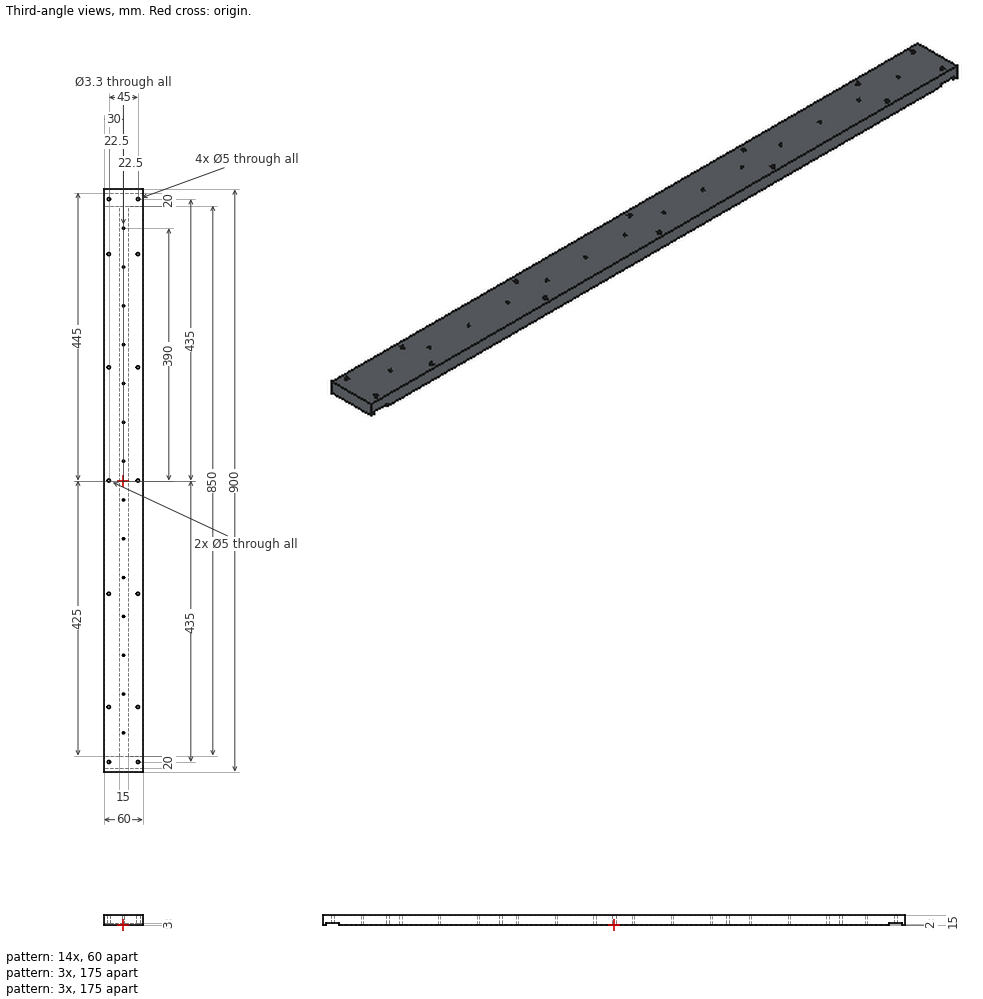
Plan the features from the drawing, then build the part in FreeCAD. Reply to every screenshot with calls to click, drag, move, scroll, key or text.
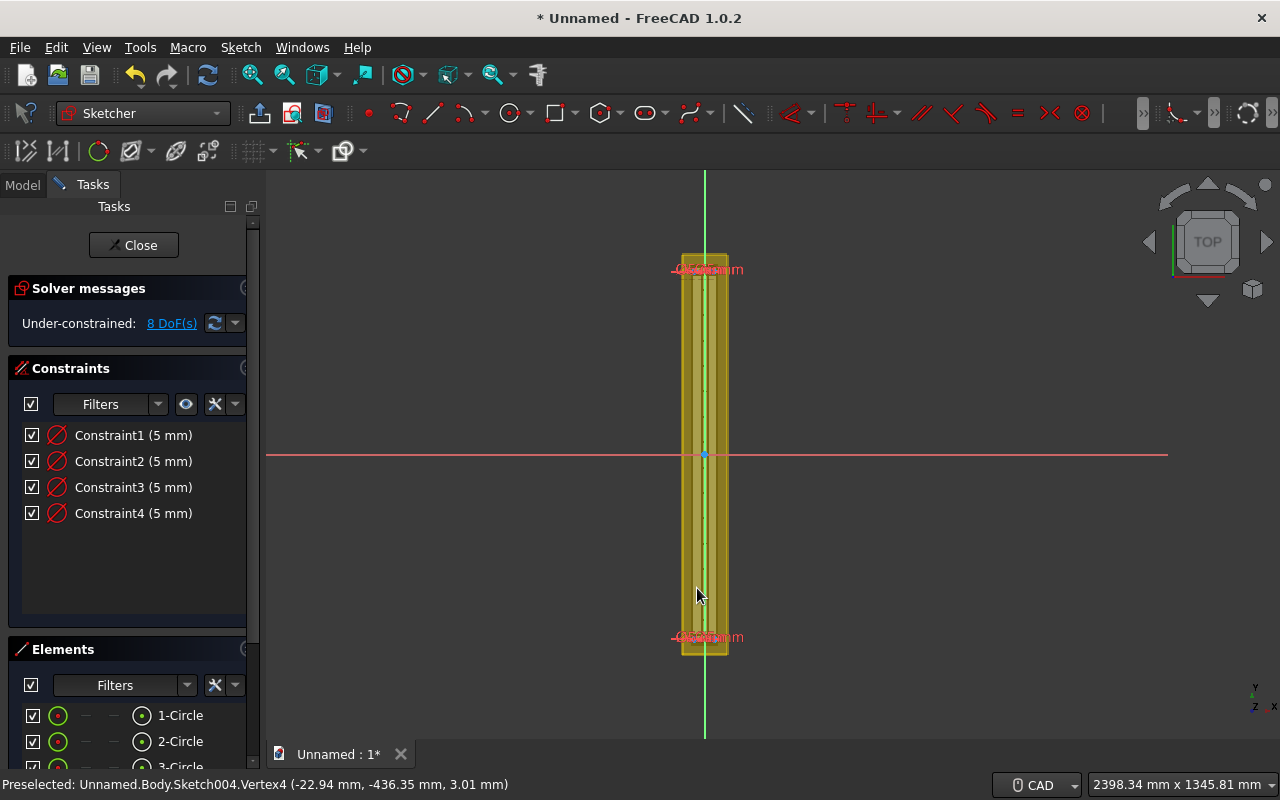
click(714, 272)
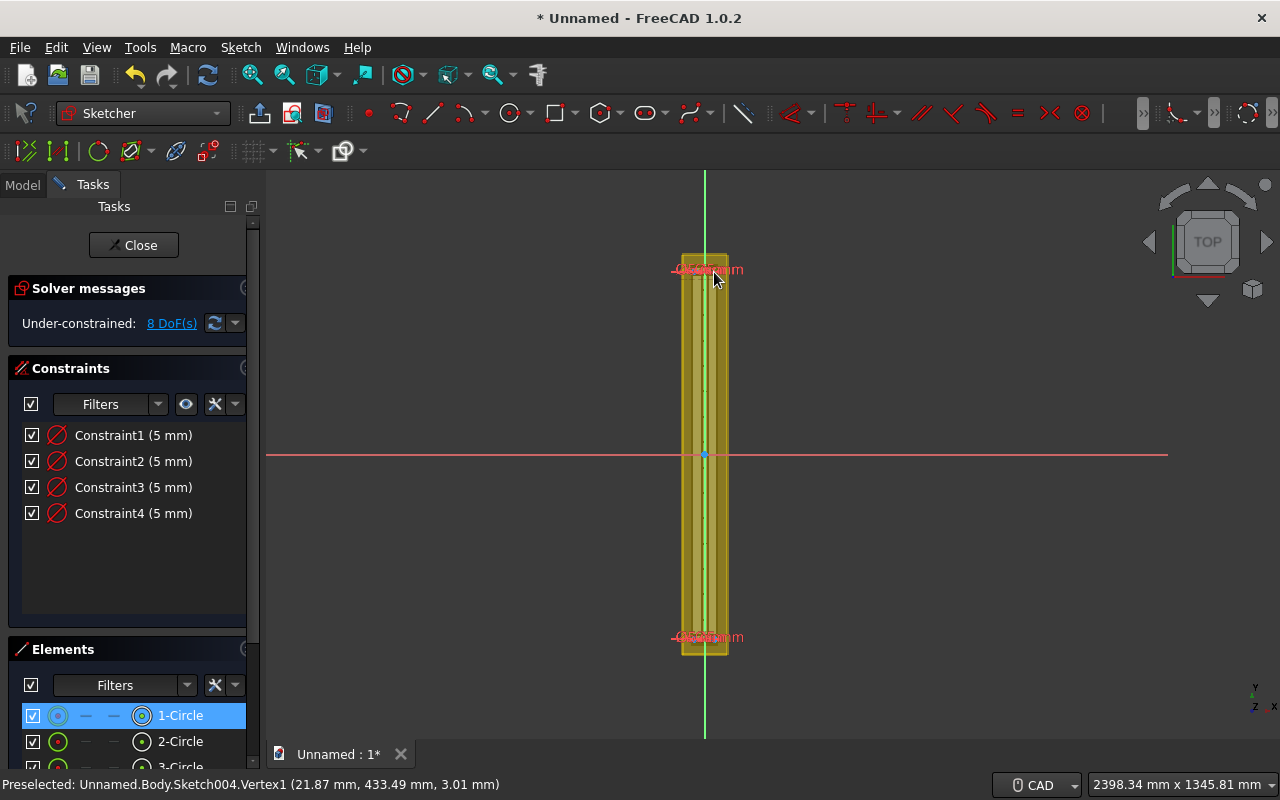
click(695, 272)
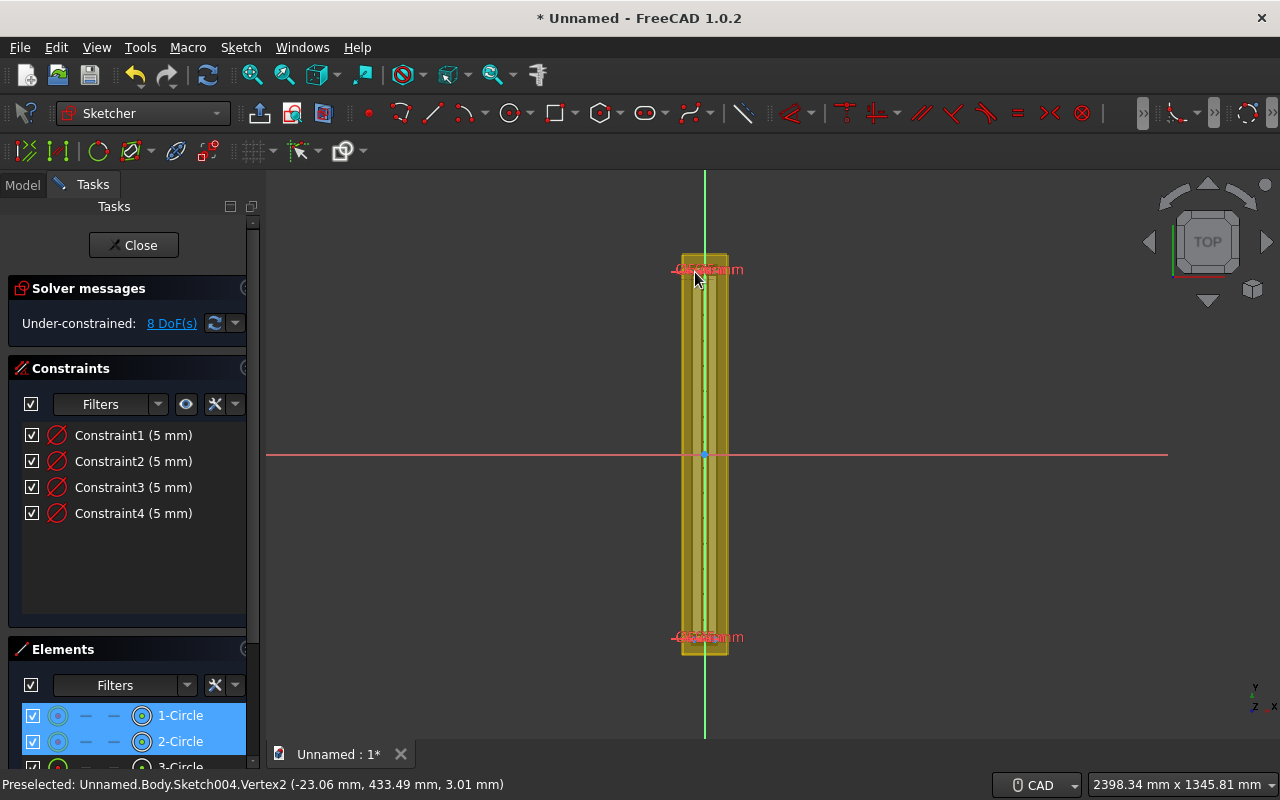
key(h)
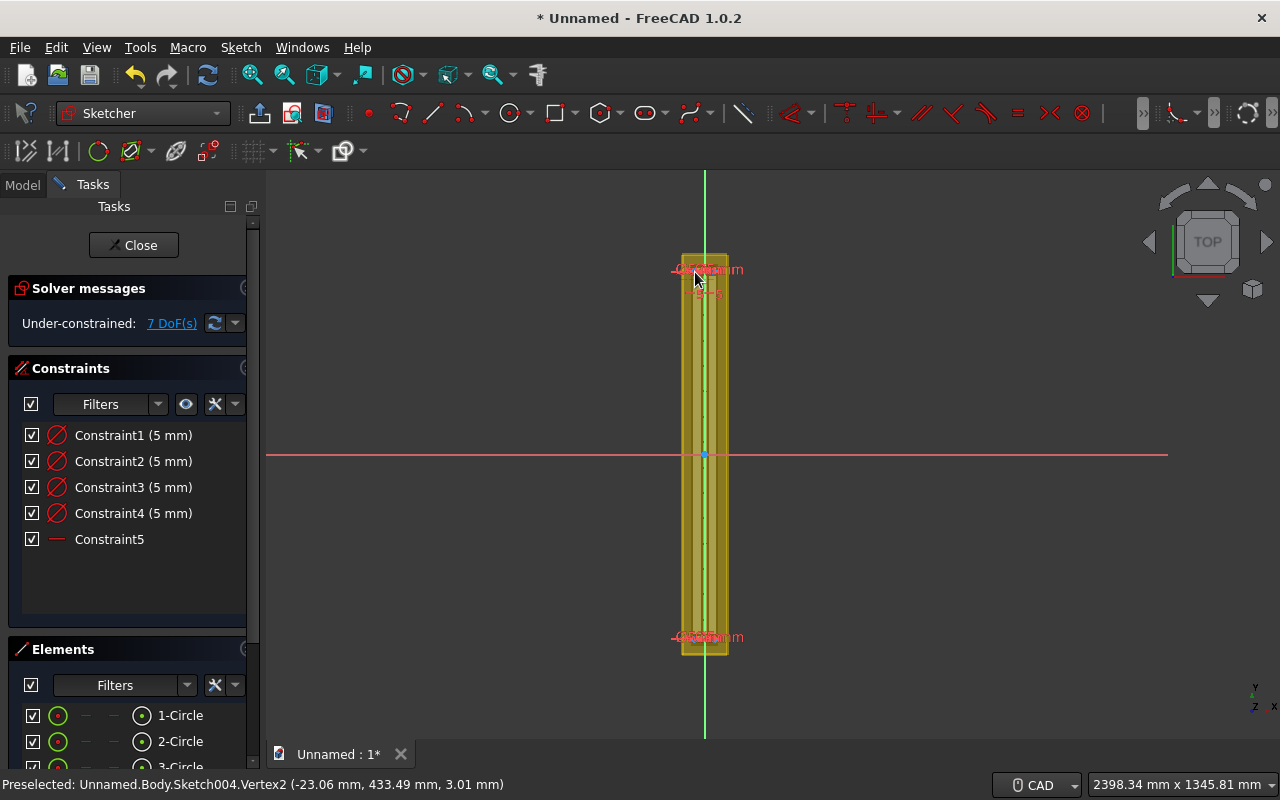
click(714, 272)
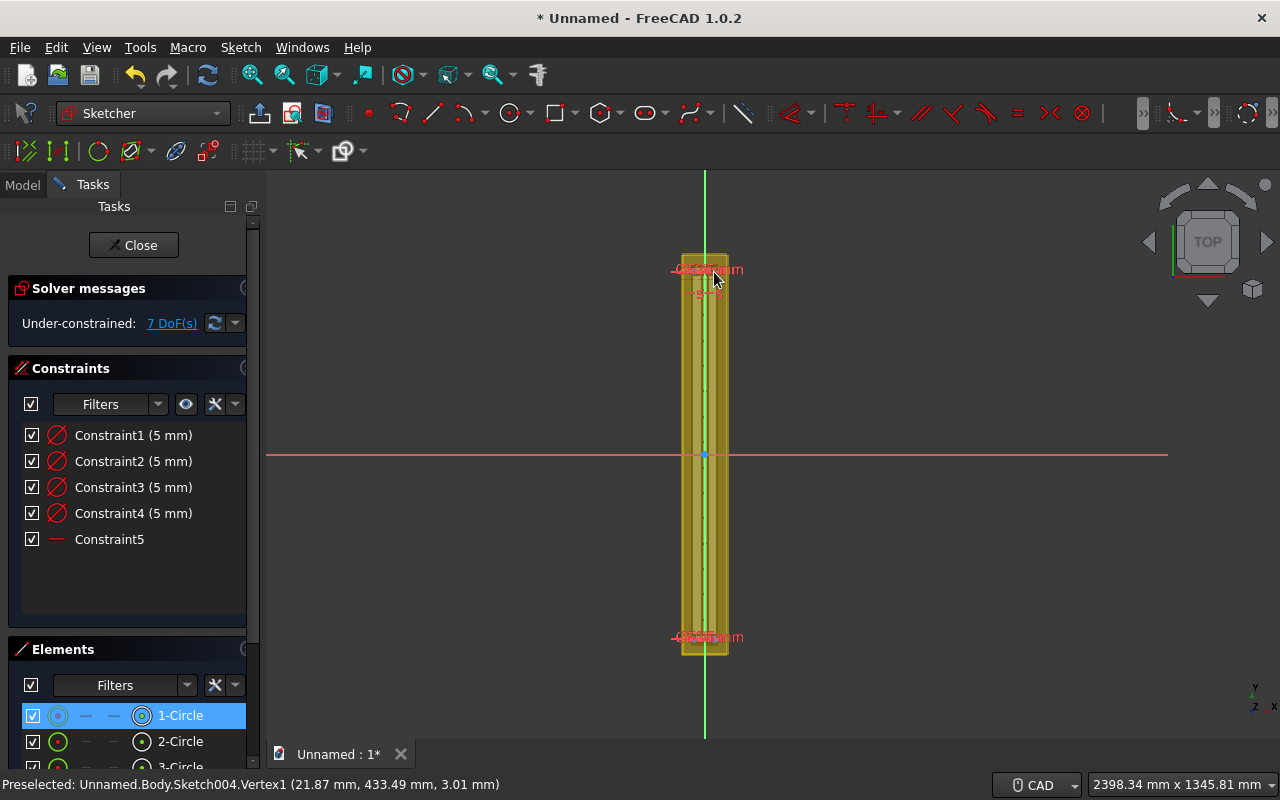
click(714, 639)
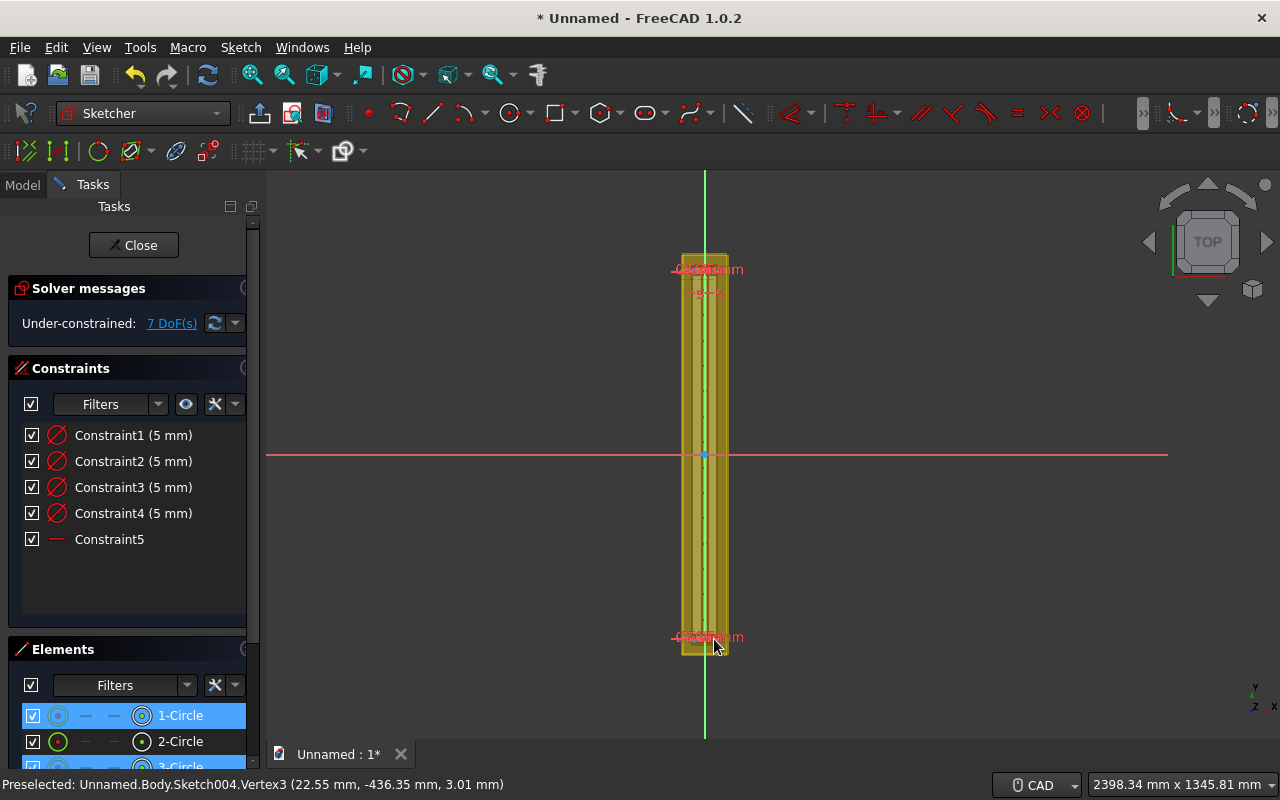
key(v)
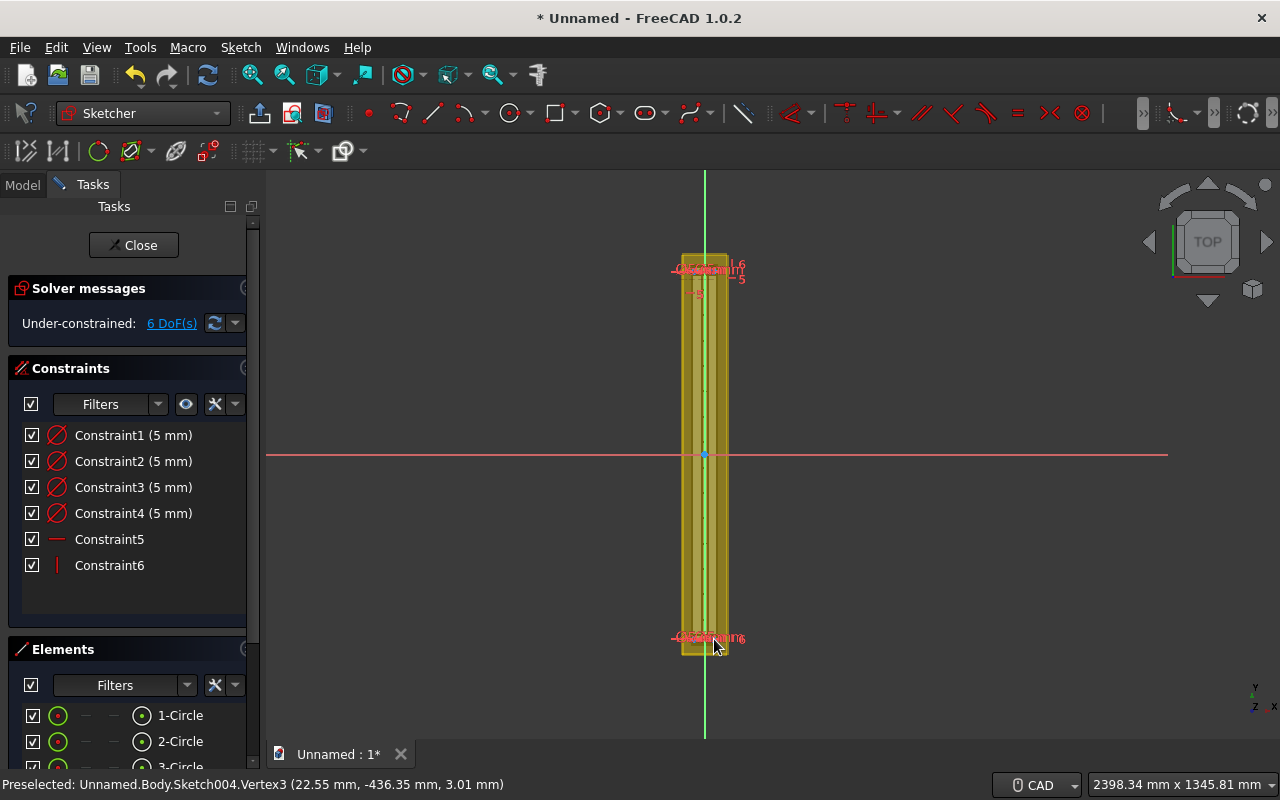
click(695, 272)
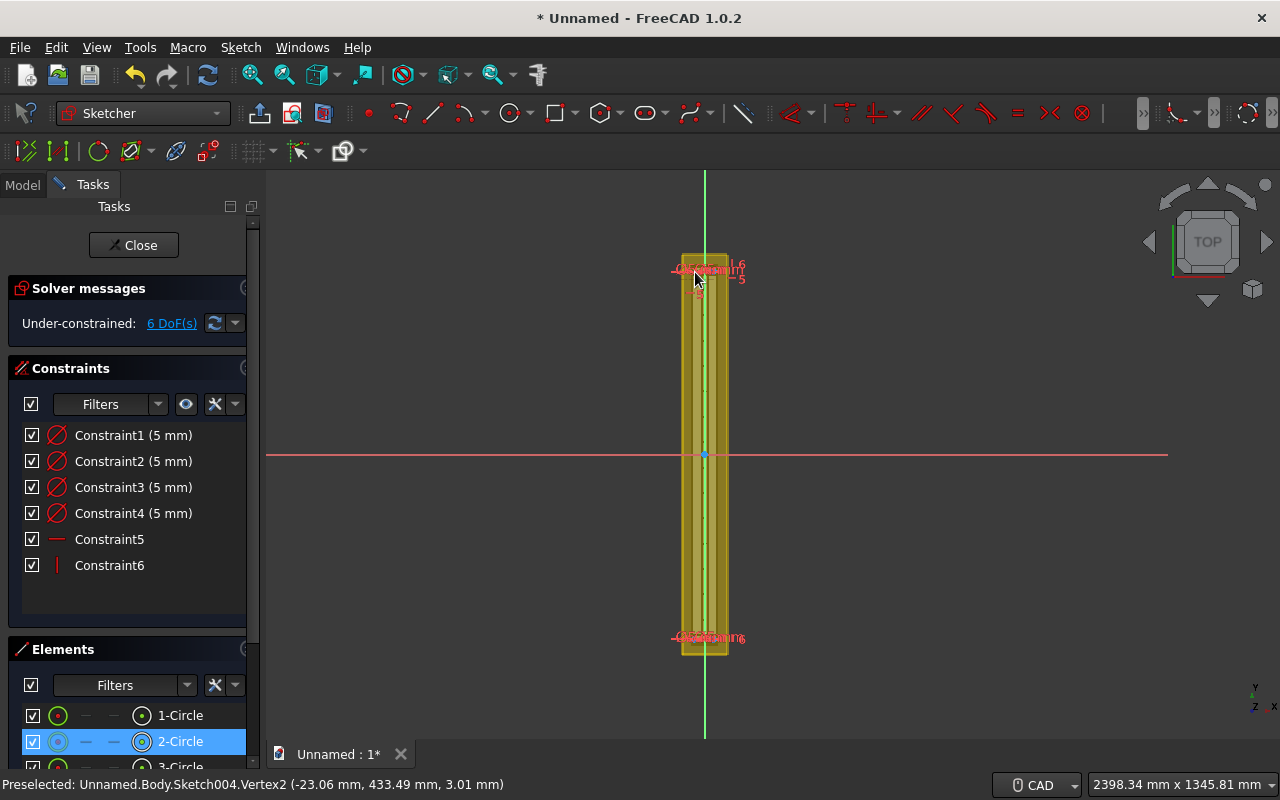
click(695, 639)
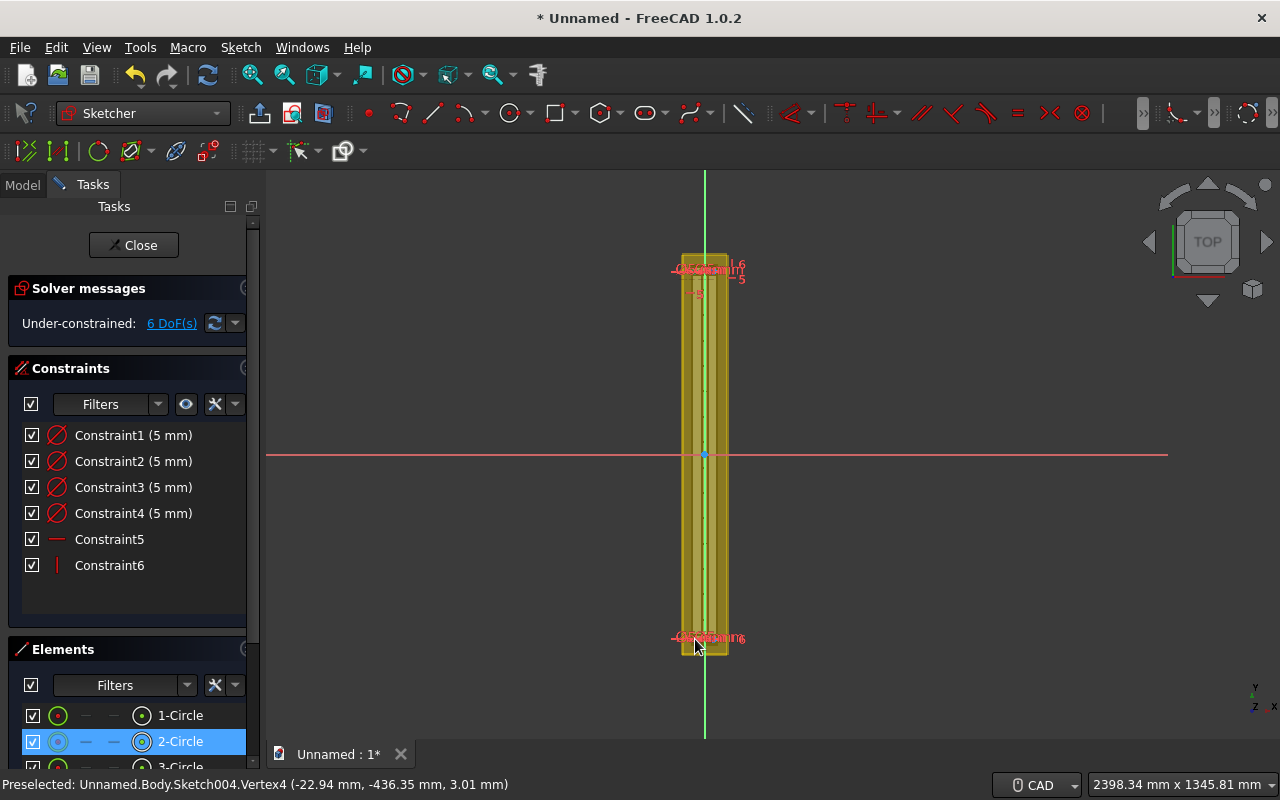
key(v)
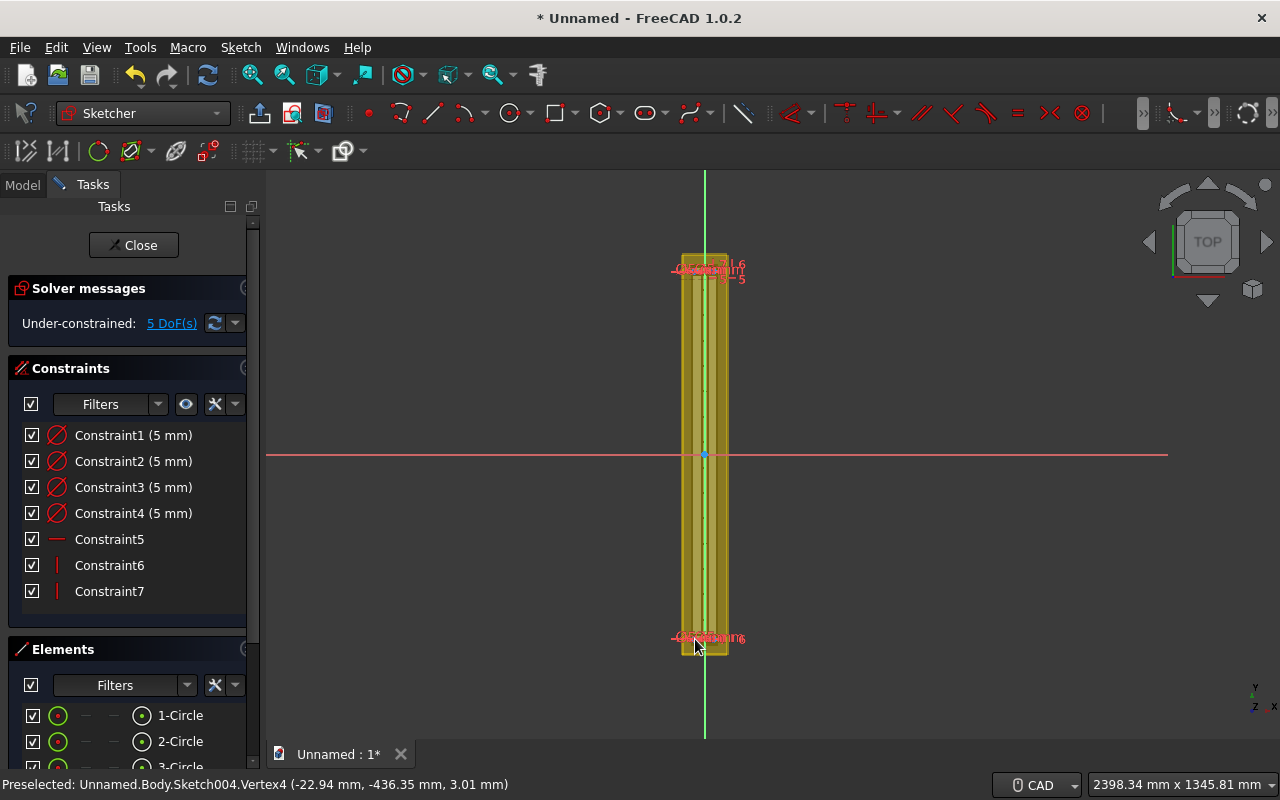
scroll(714, 639, up, 4)